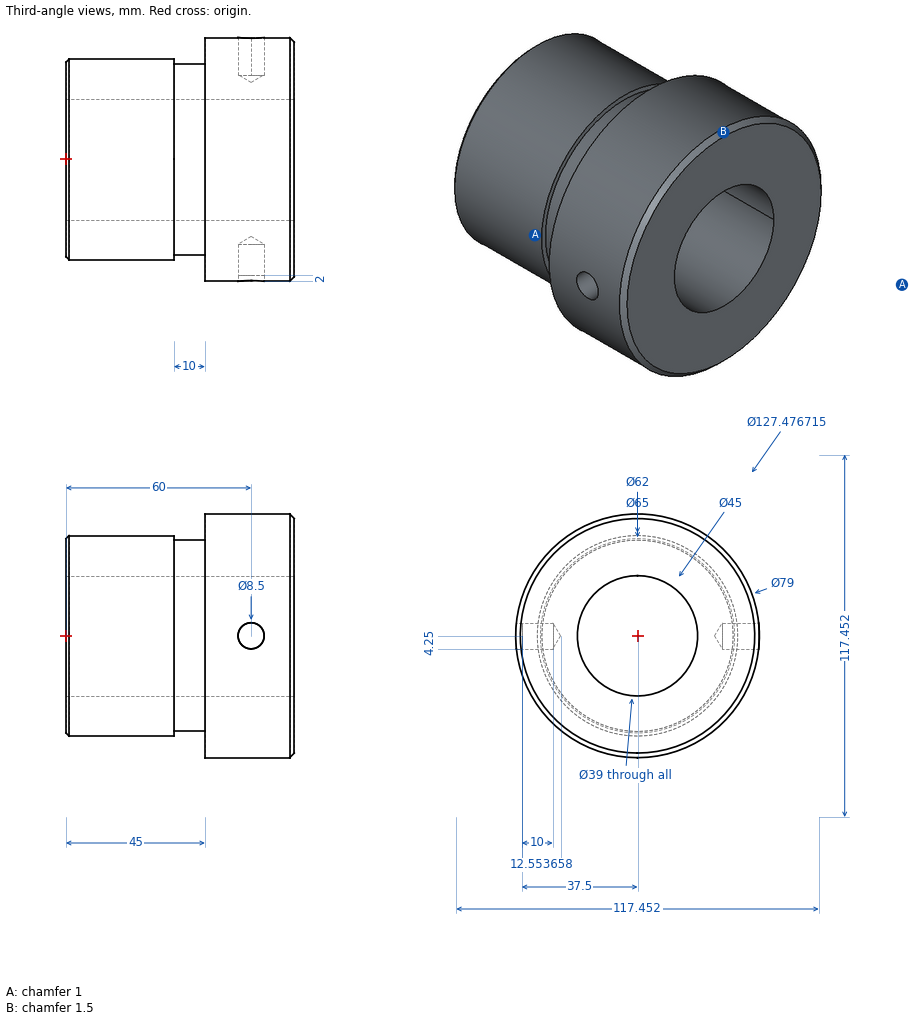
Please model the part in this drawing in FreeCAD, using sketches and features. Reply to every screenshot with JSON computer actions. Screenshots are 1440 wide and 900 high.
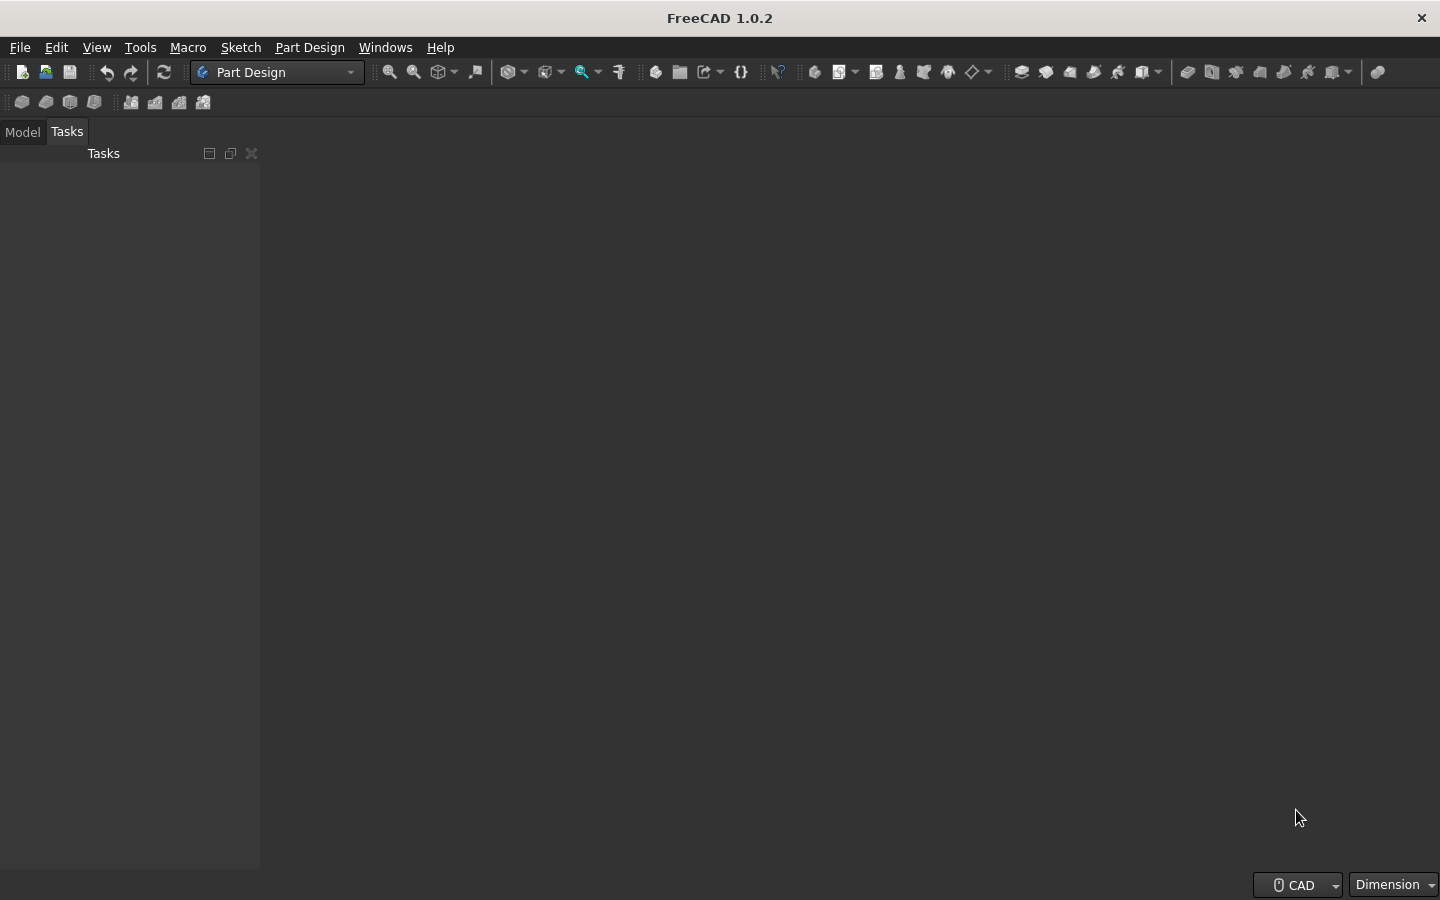
{"action": "left_click", "coordinate": [22, 72]}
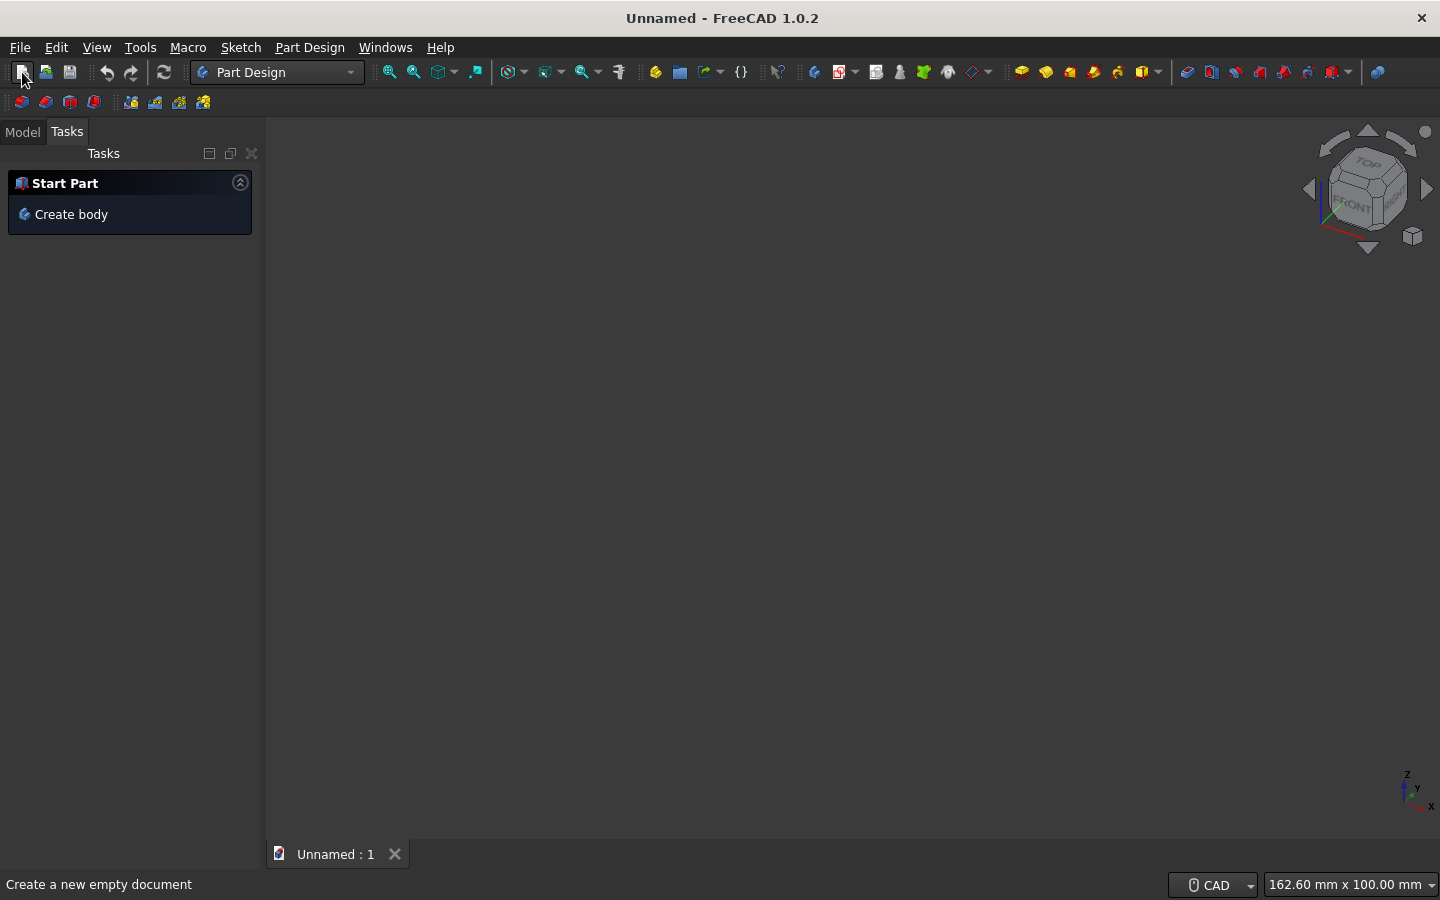
{"action": "left_click", "coordinate": [840, 72]}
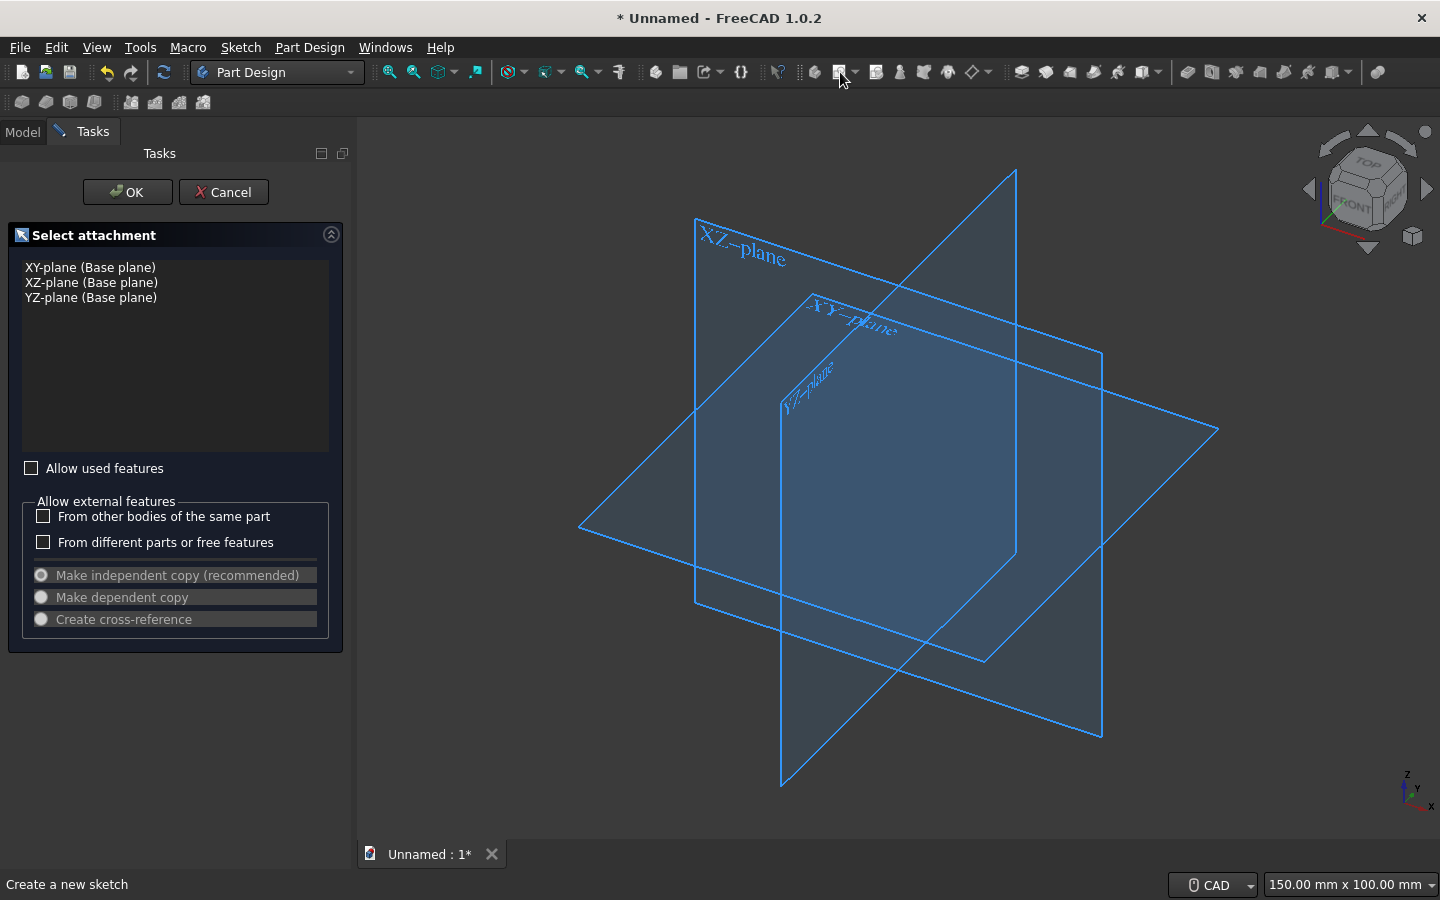
{"action": "left_click", "coordinate": [82, 298]}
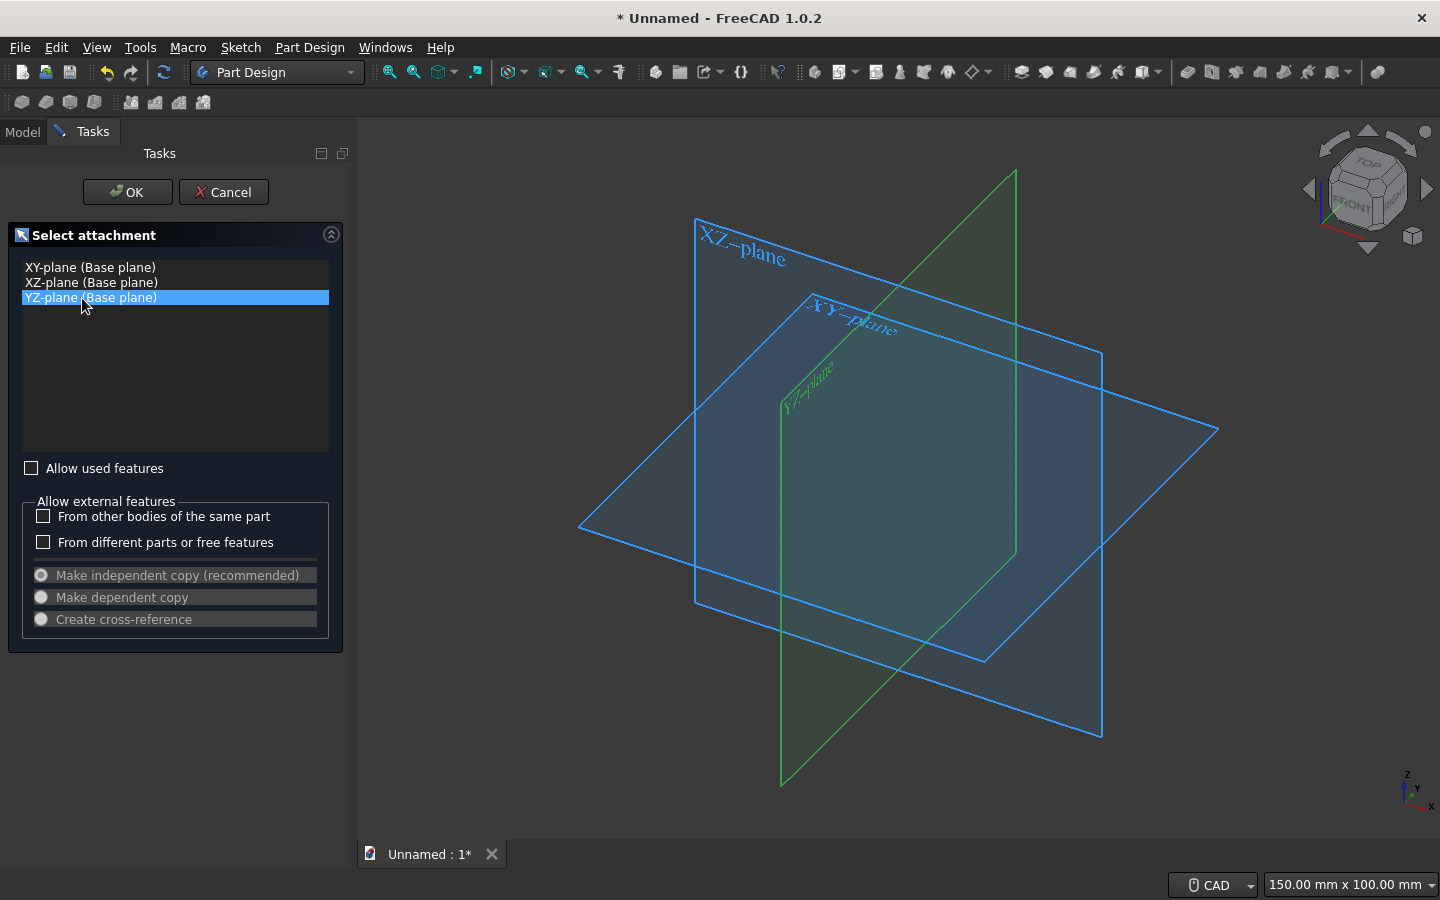
{"action": "left_click", "coordinate": [128, 192]}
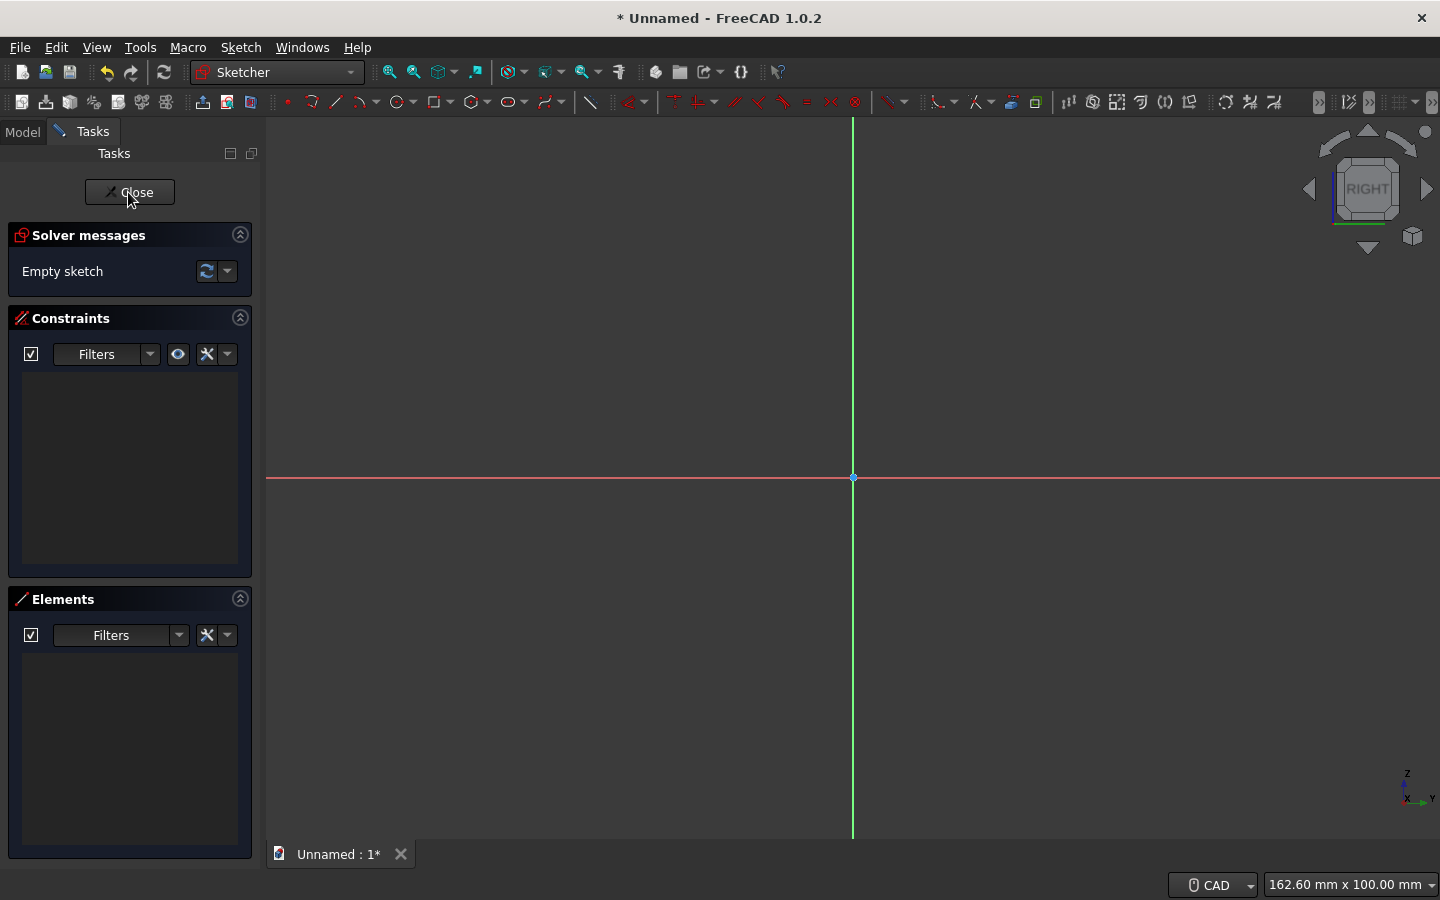
{"action": "key", "text": "g c"}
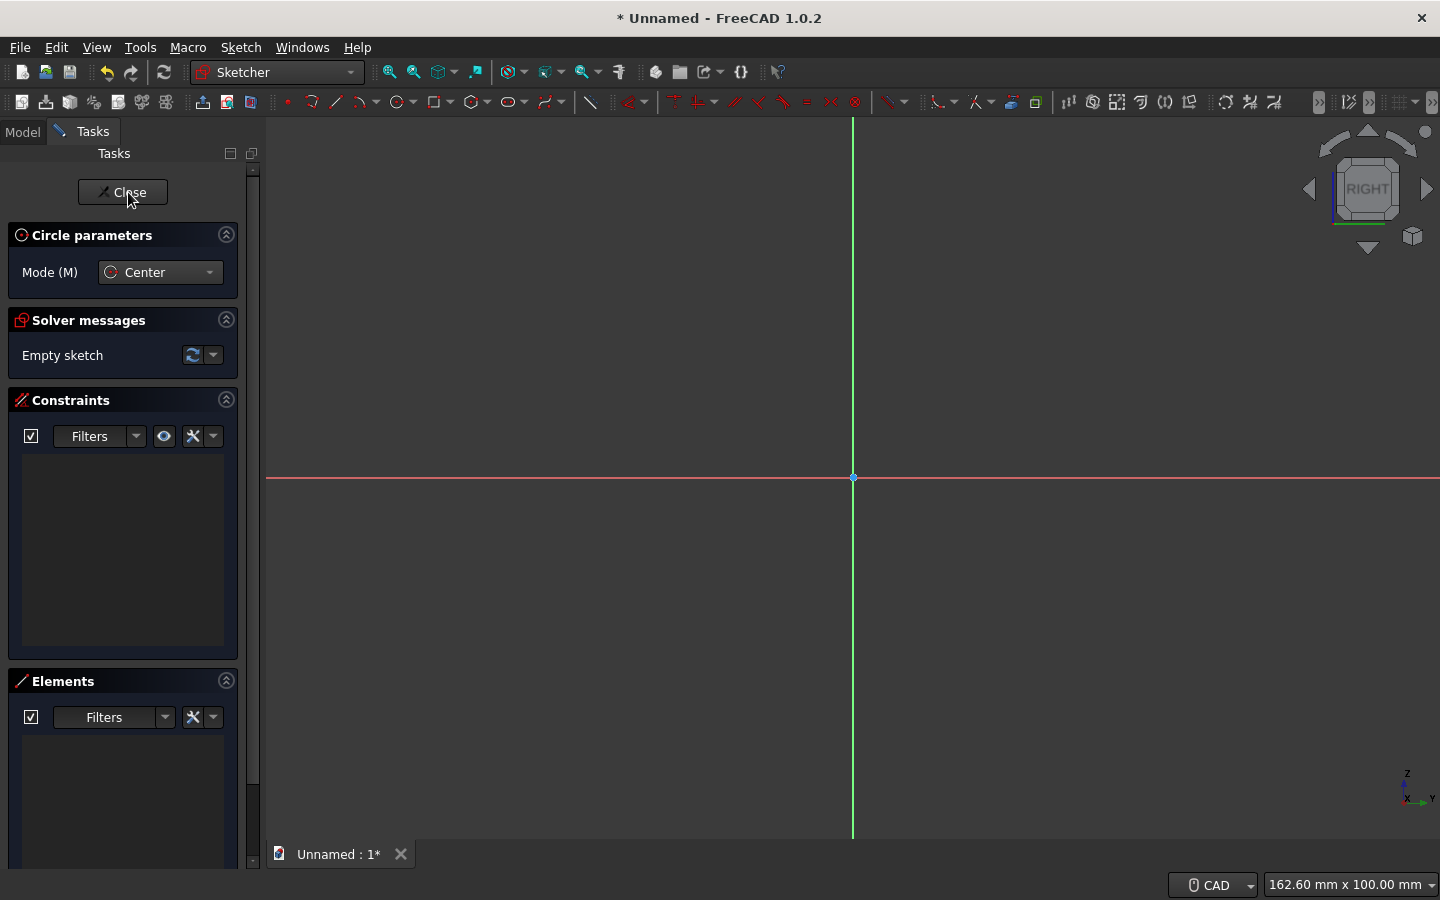
{"action": "left_click", "coordinate": [853, 478]}
{"action": "mouse_move", "coordinate": [1055, 276]}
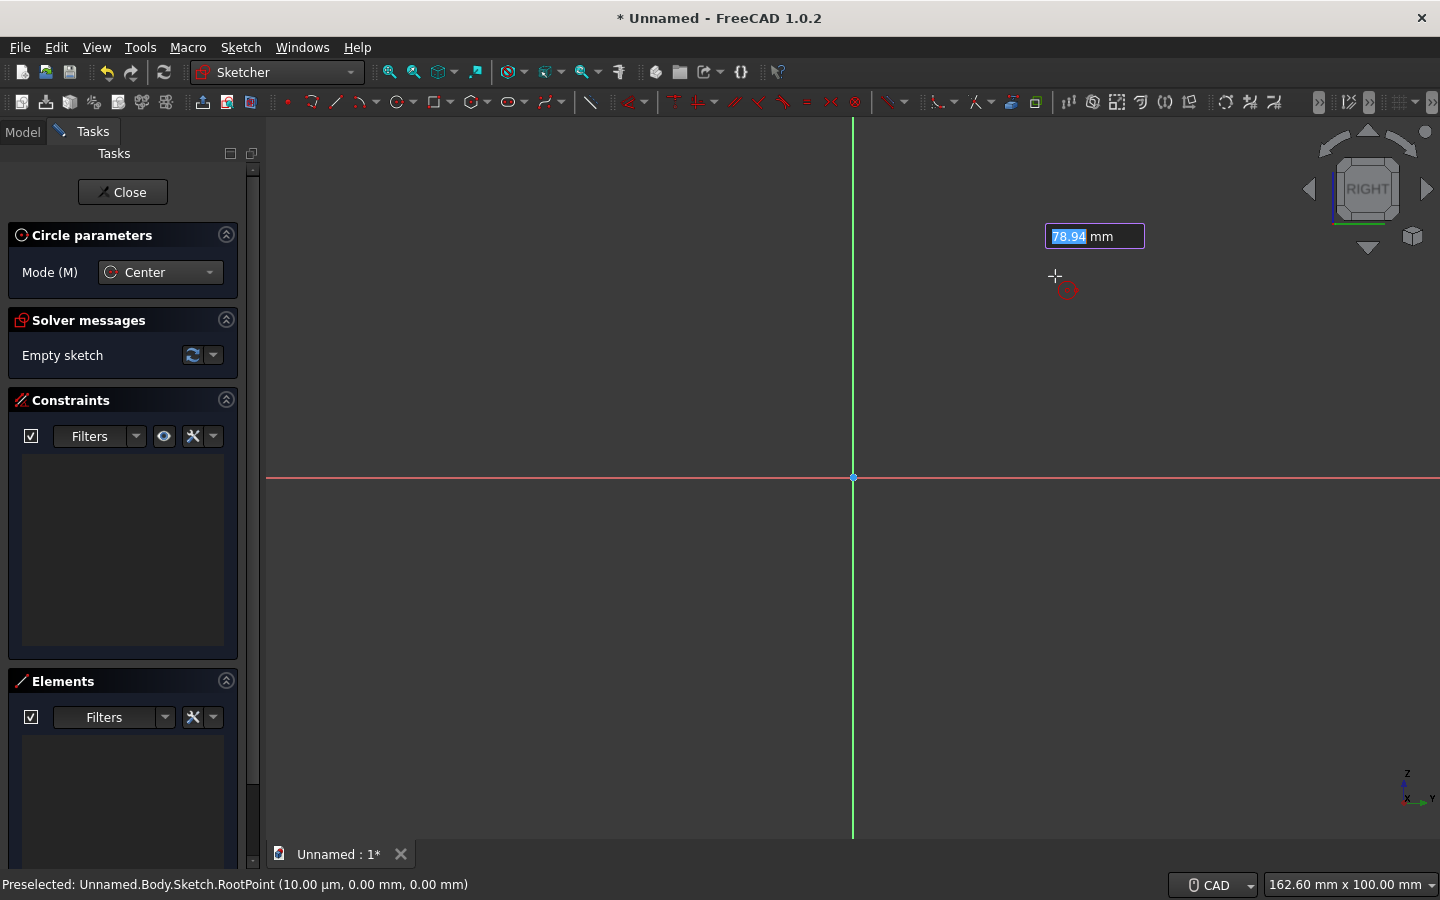
{"action": "type", "text": "79"}
{"action": "key", "text": "Return"}
{"action": "key", "text": "Escape"}